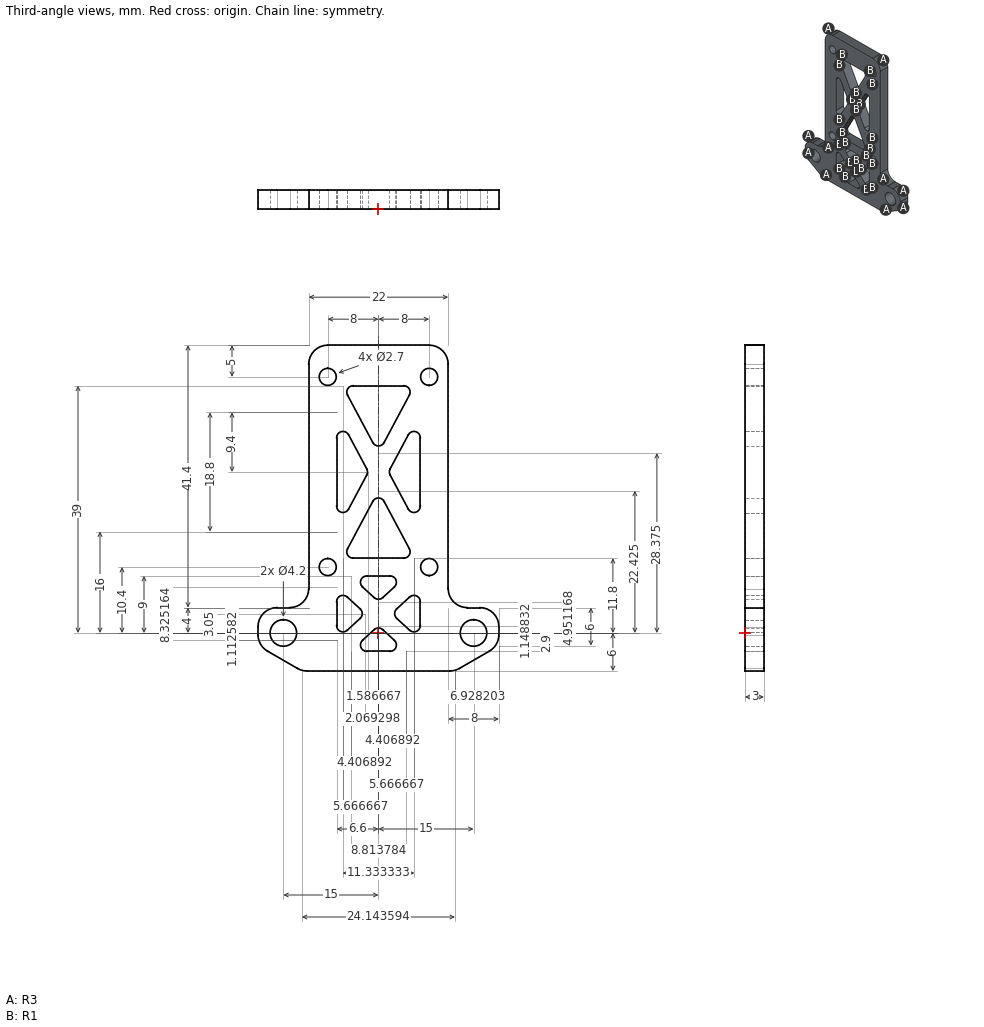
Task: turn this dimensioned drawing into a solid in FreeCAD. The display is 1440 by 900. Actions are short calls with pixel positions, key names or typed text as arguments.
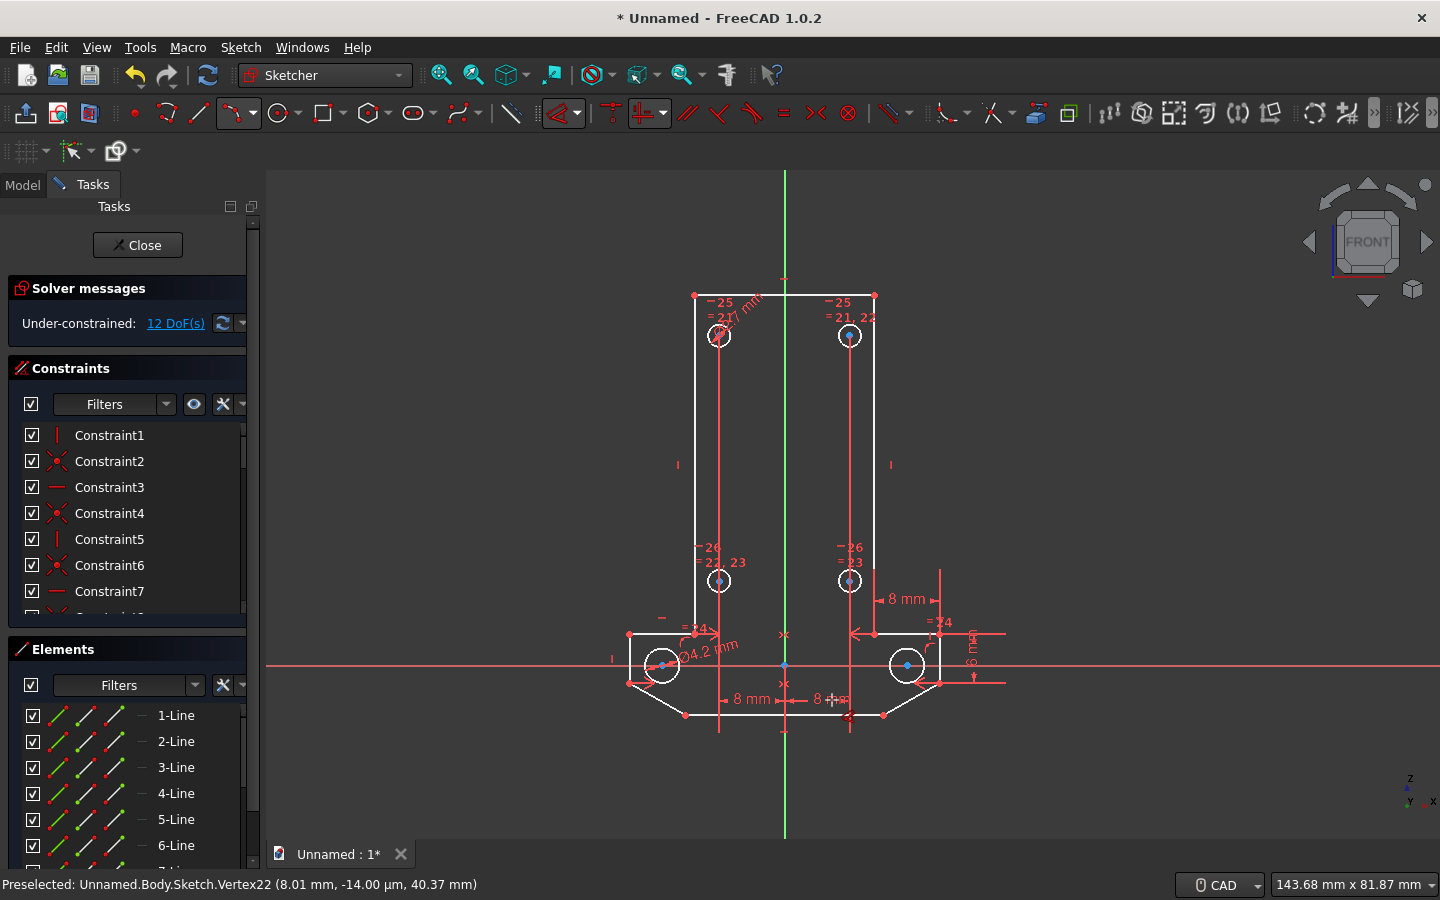
click(719, 581)
click(752, 547)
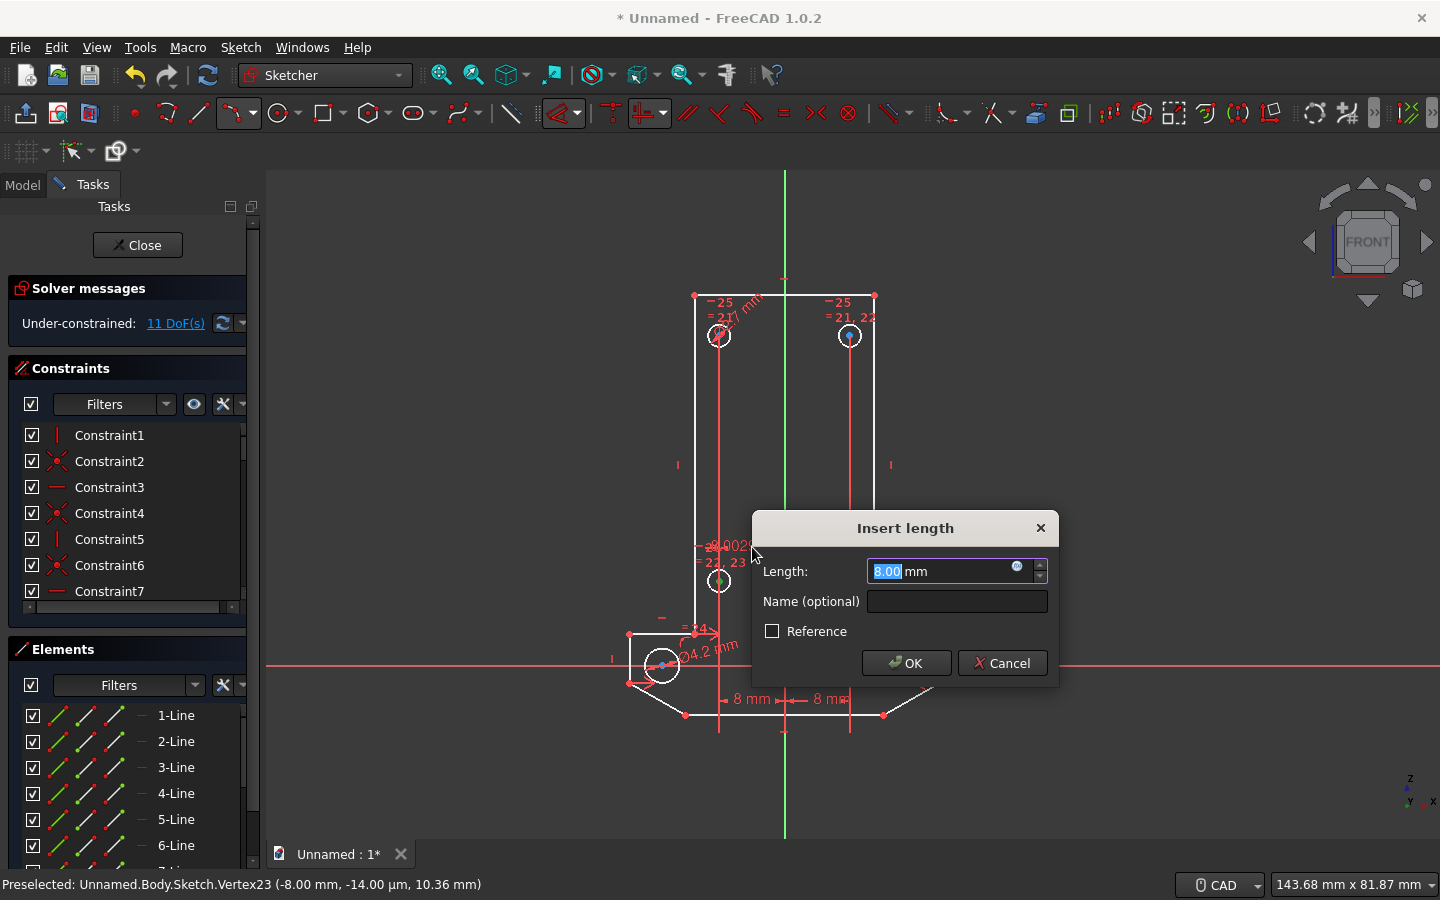
text(8)
key(Return)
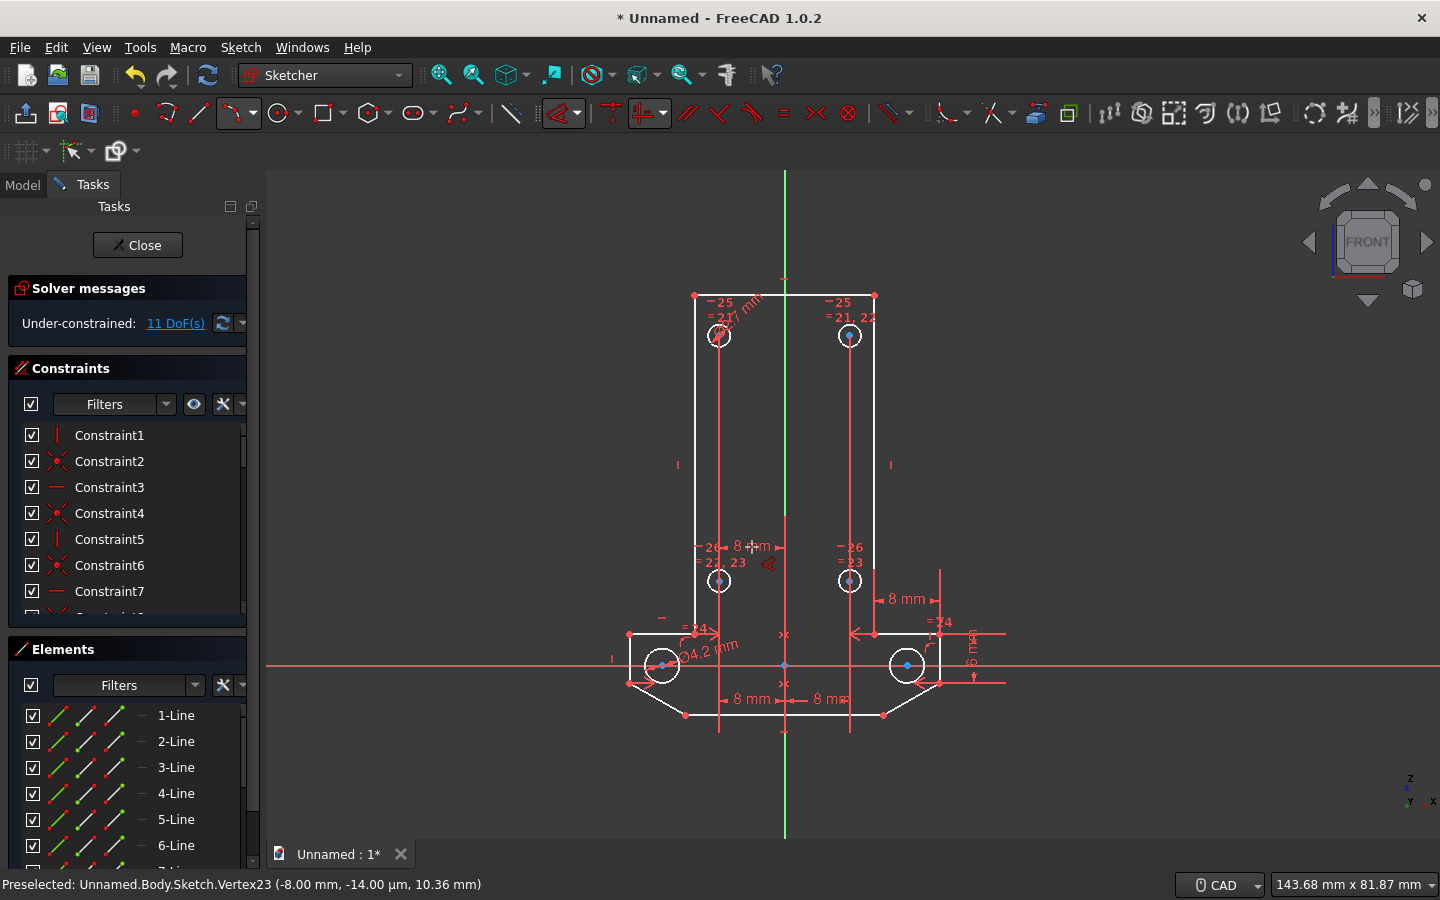
click(850, 581)
click(832, 547)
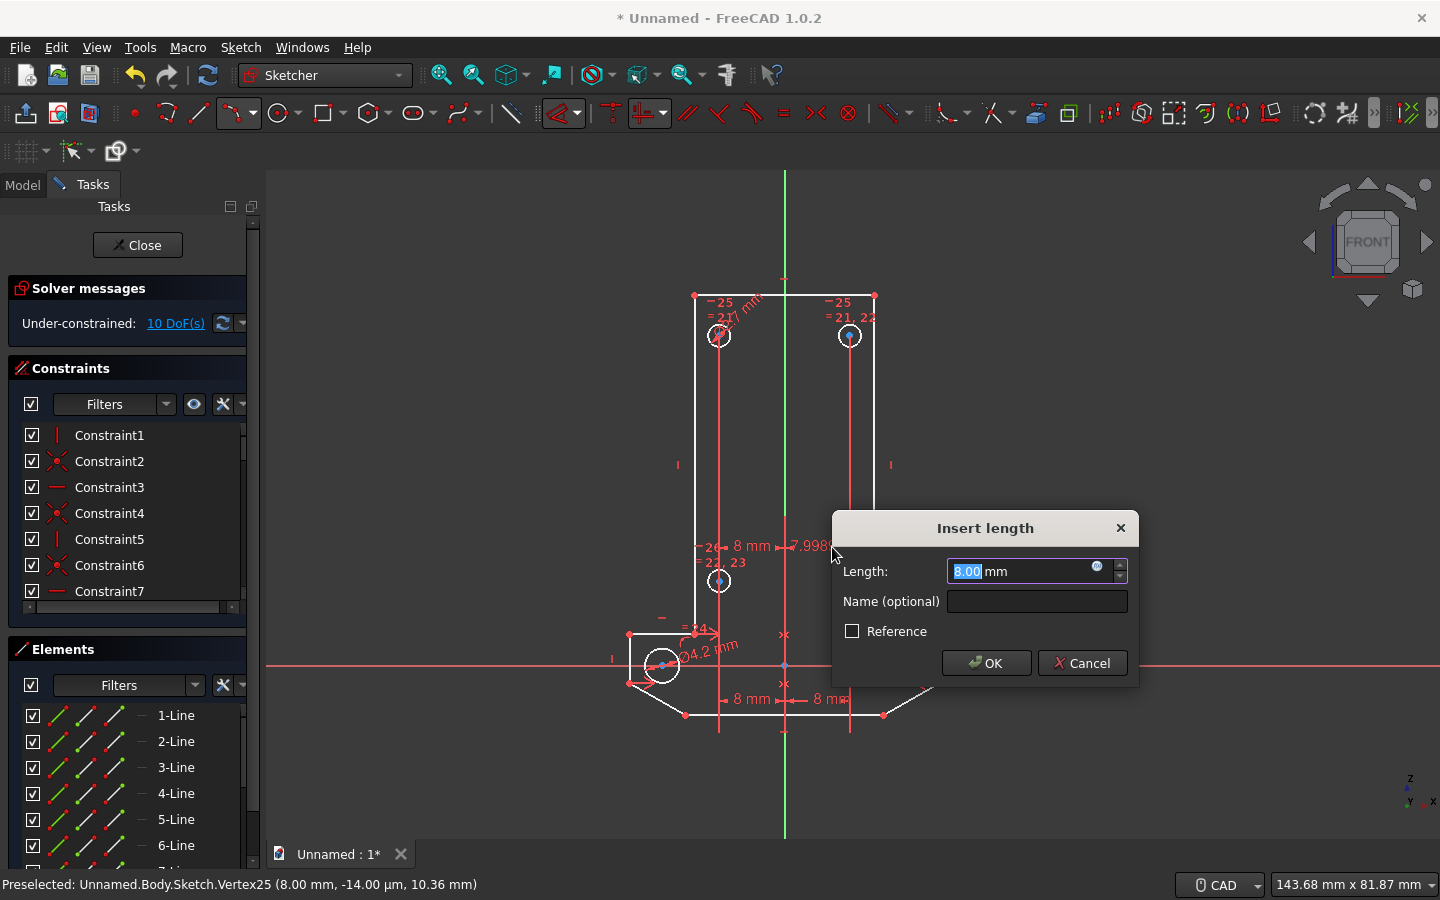
text(8)
key(Return)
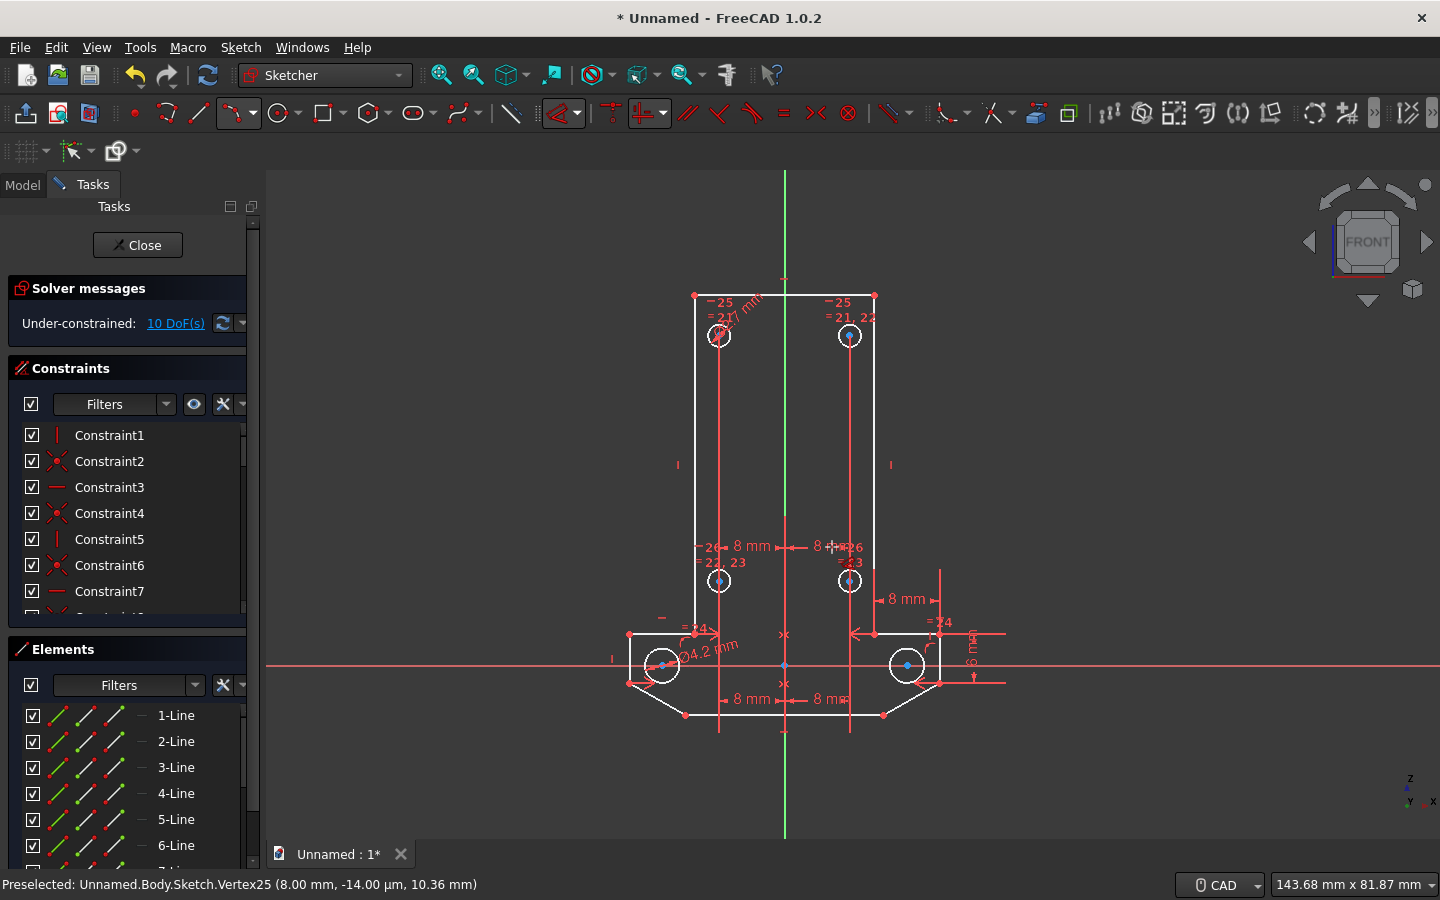
click(749, 295)
click(743, 261)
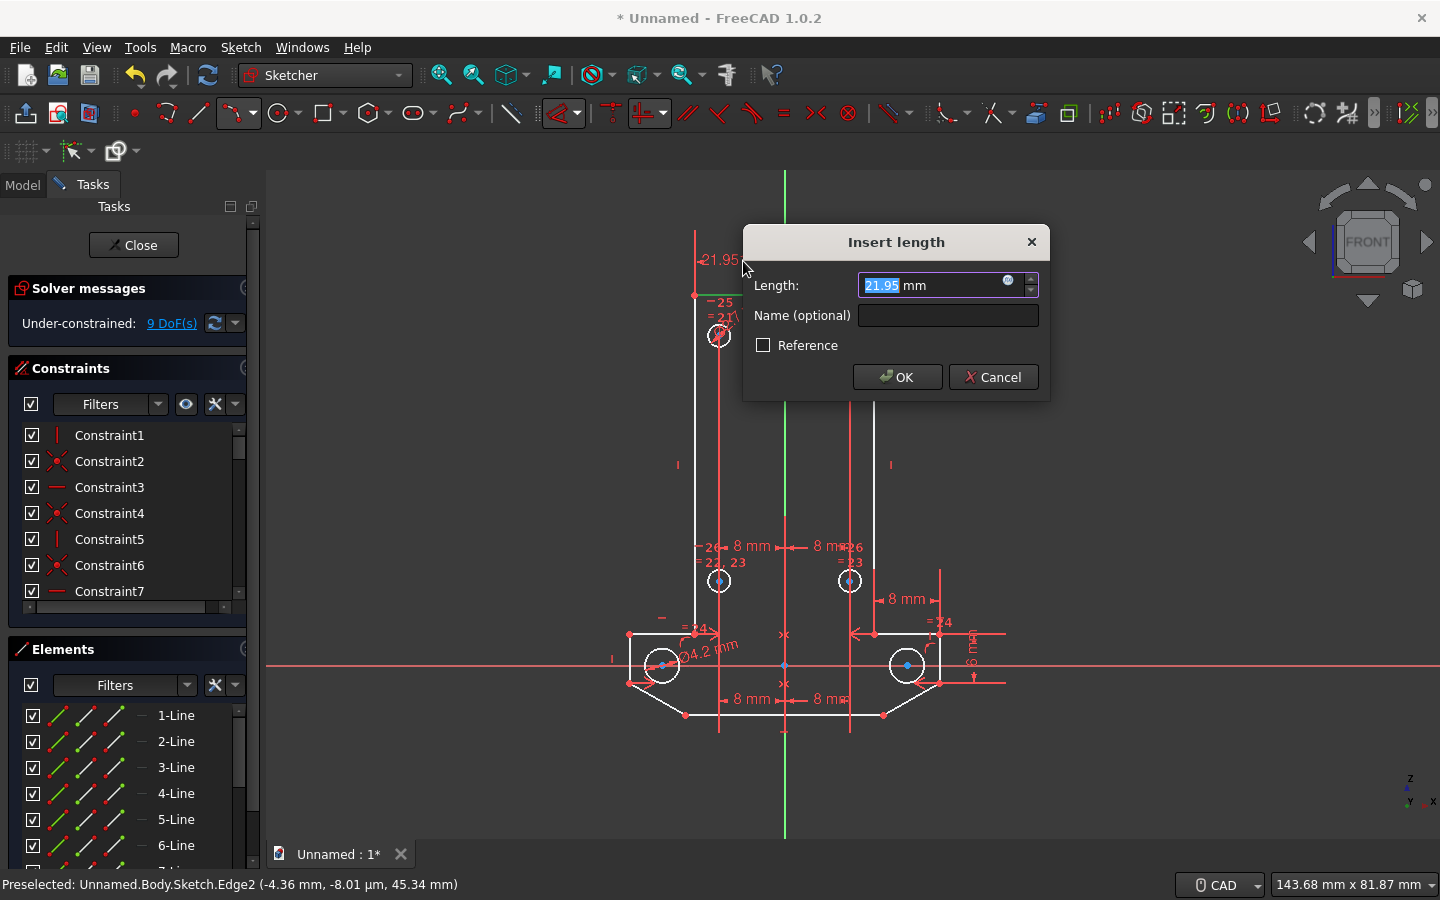
text(22)
key(Return)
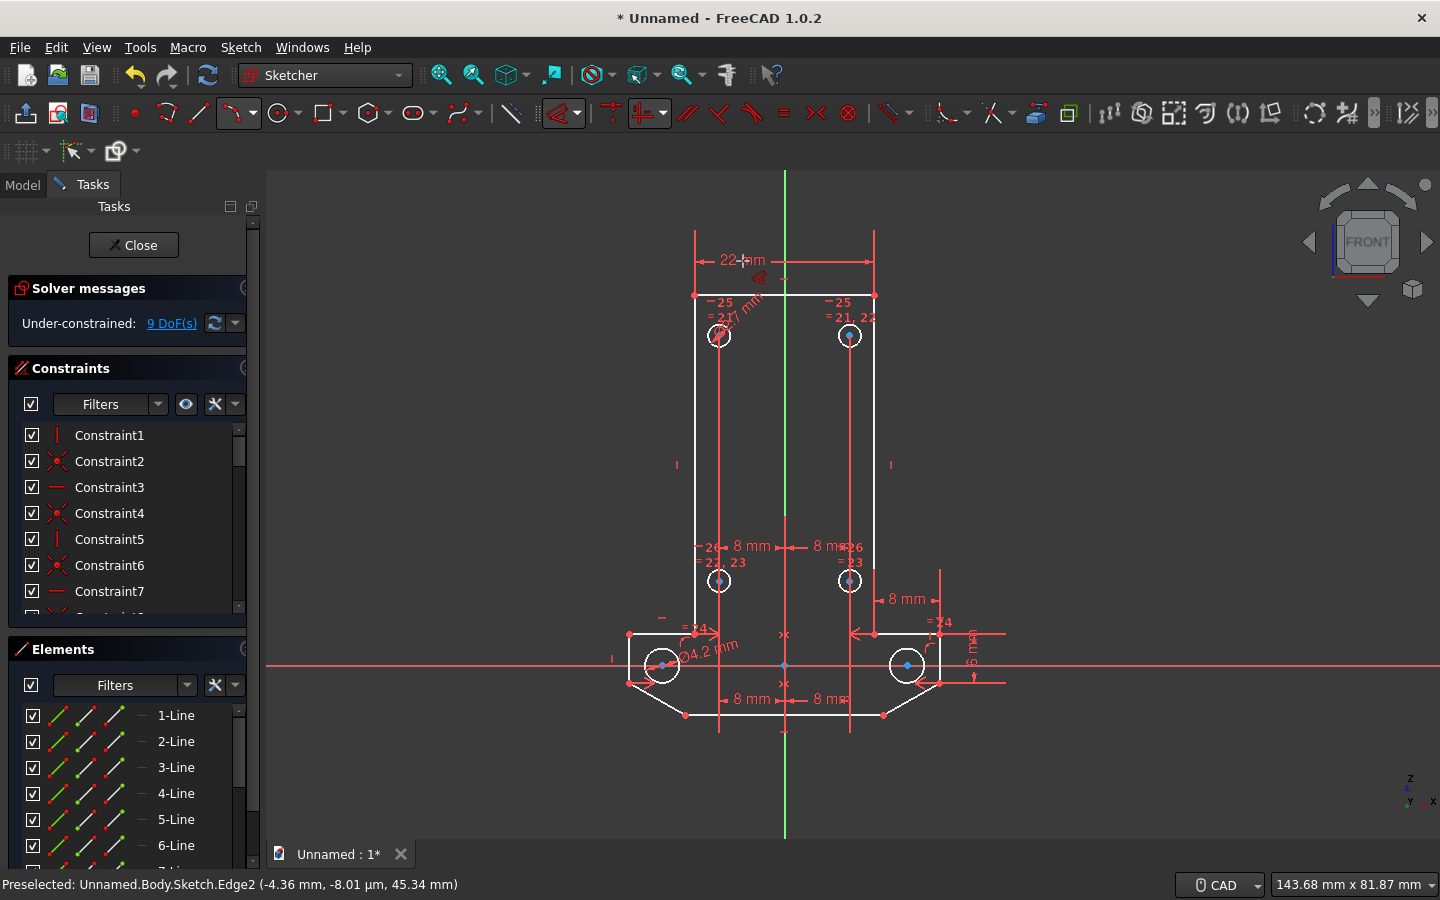
click(695, 634)
click(819, 650)